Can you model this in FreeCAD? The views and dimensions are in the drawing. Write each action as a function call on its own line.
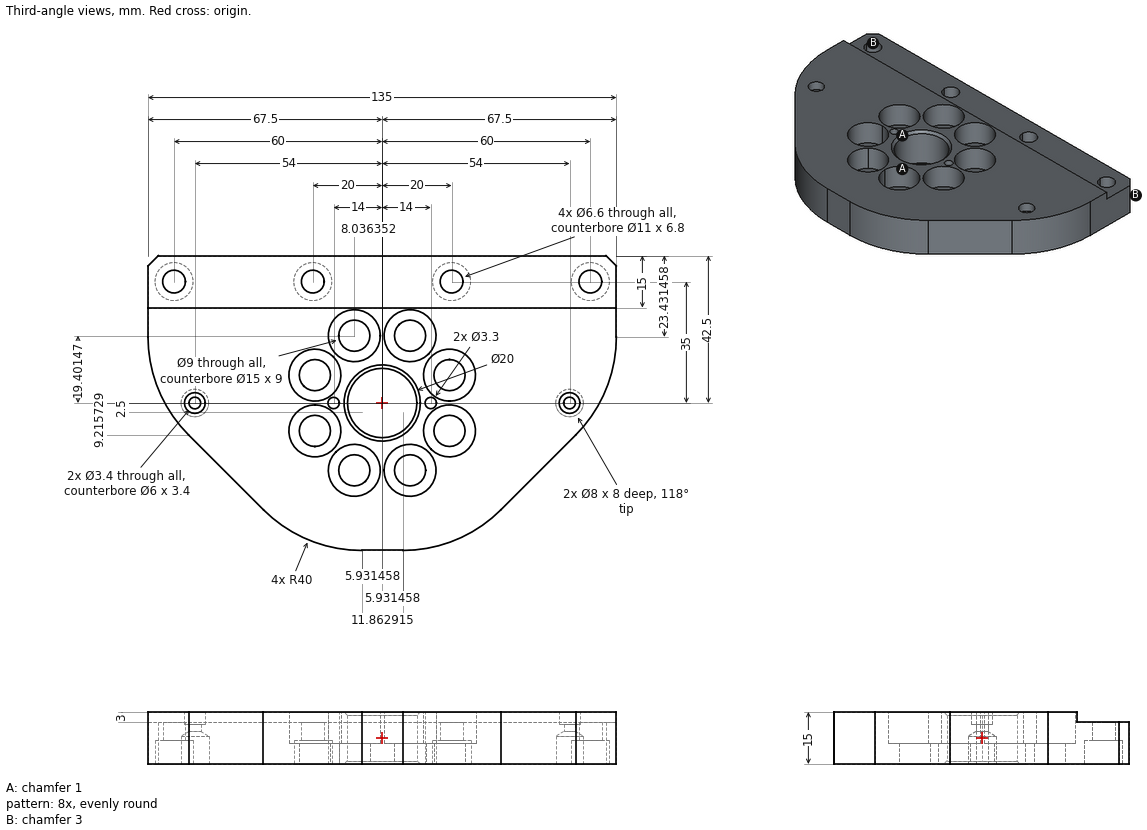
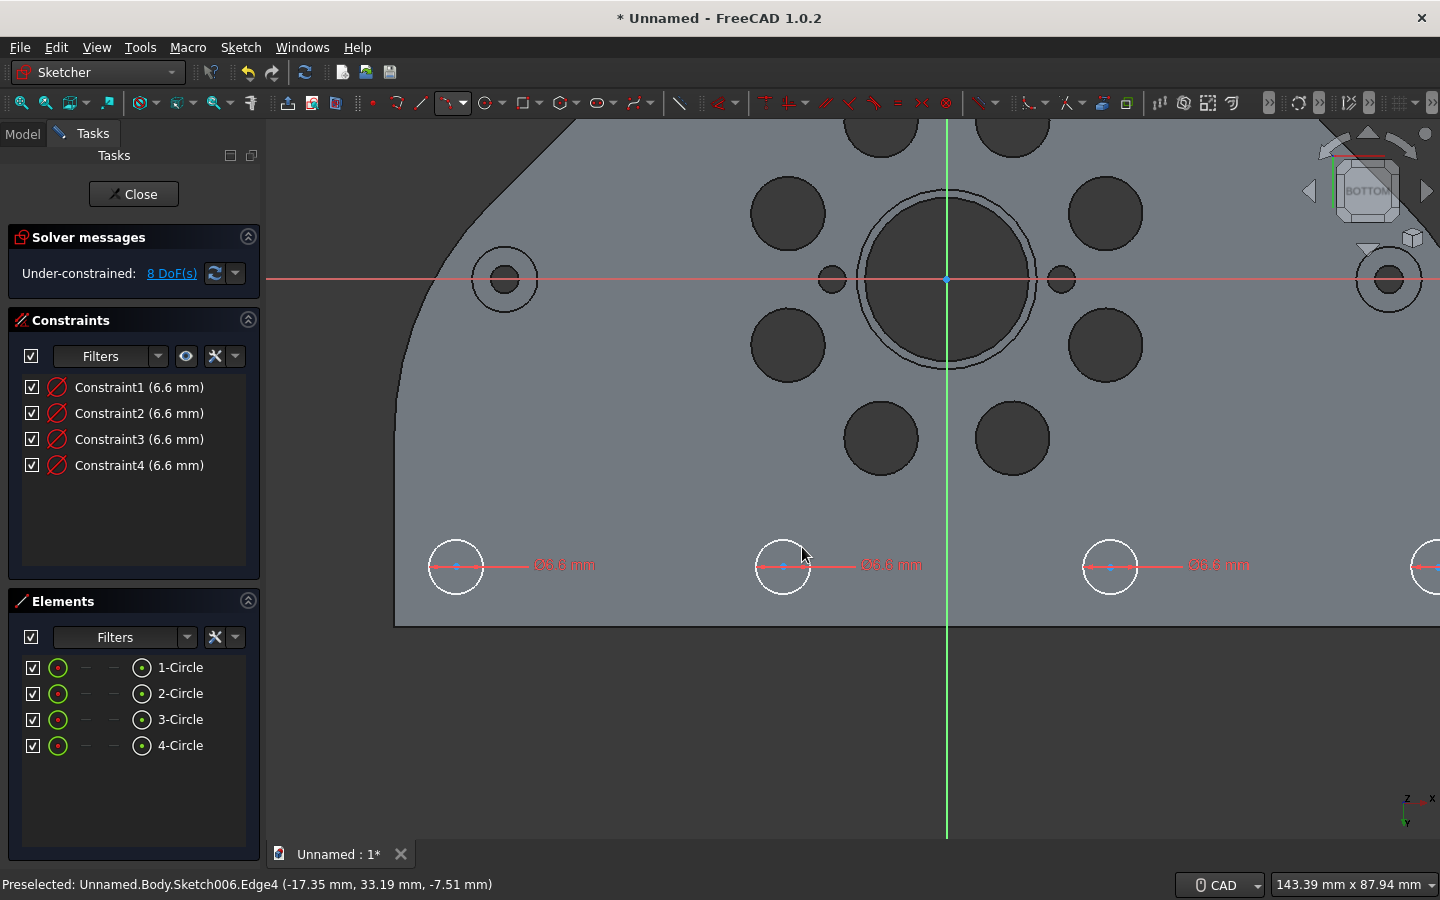
click(1110, 567)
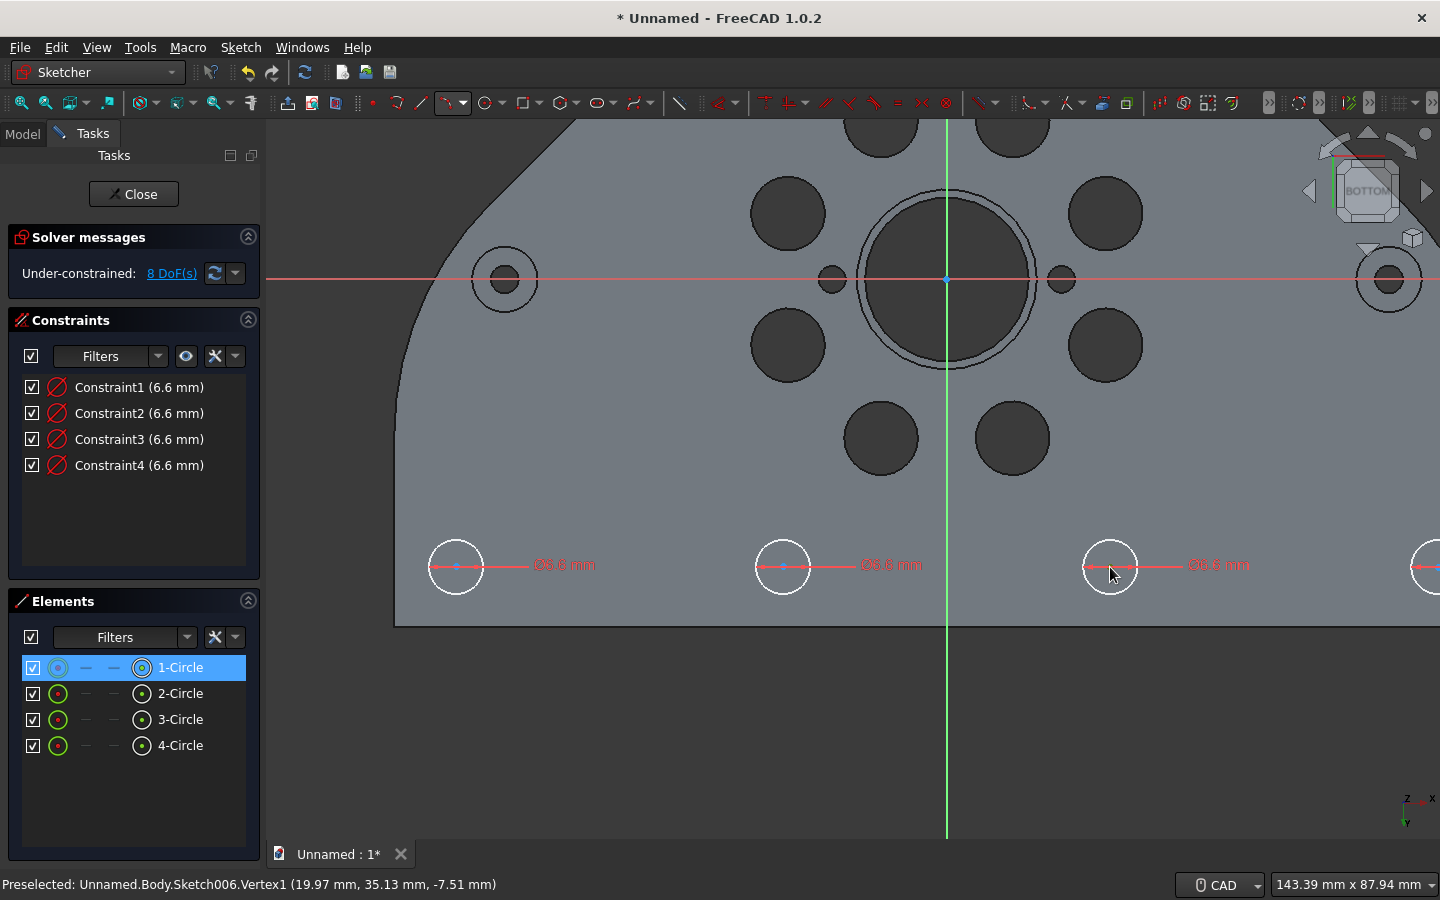
scroll(454, 566, down, 2)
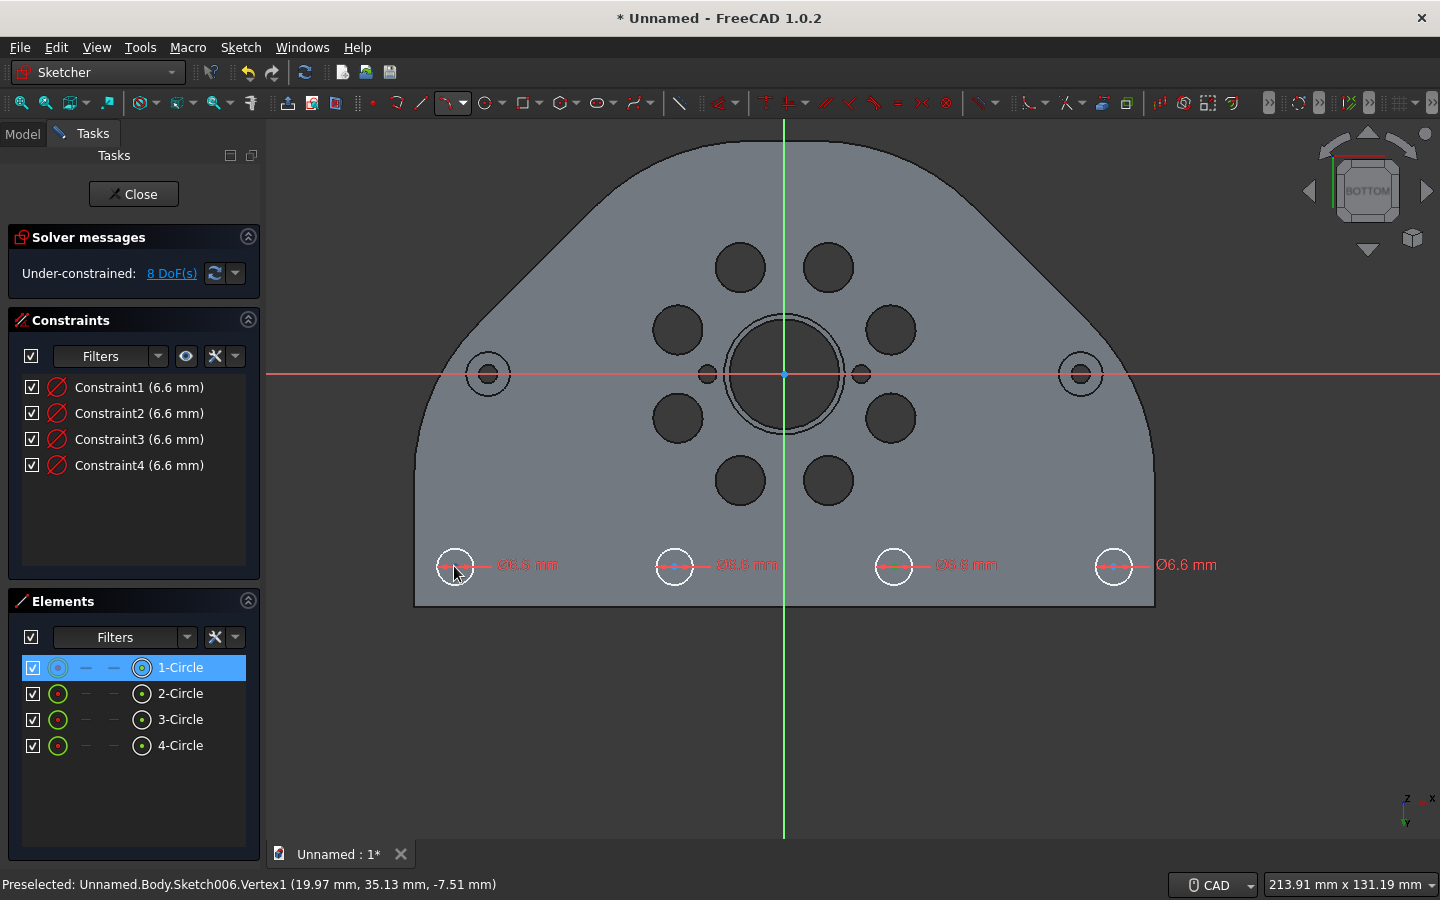
click(1114, 567)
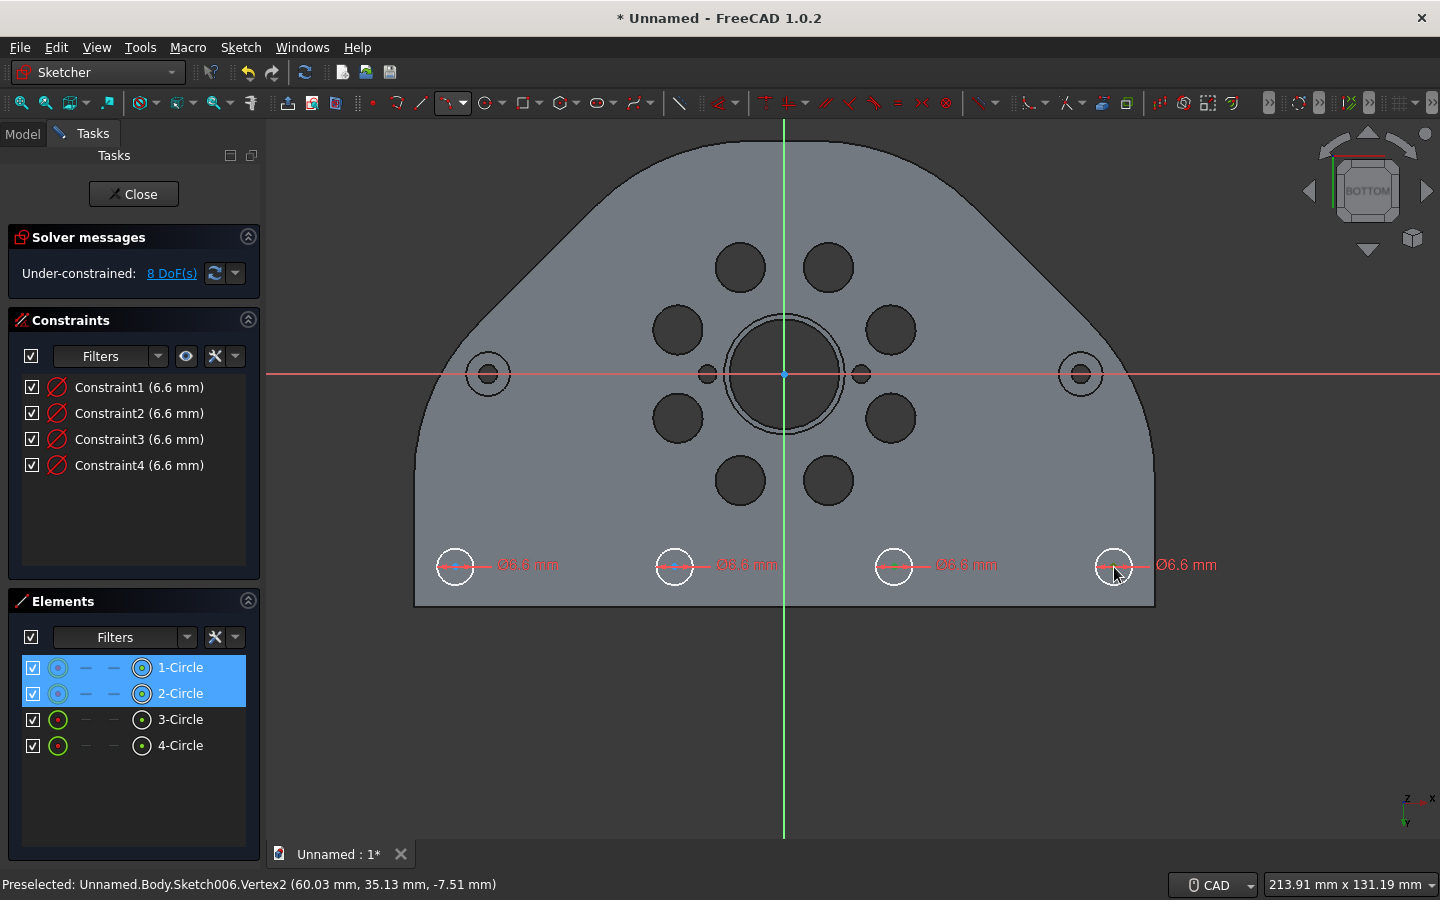
click(808, 104)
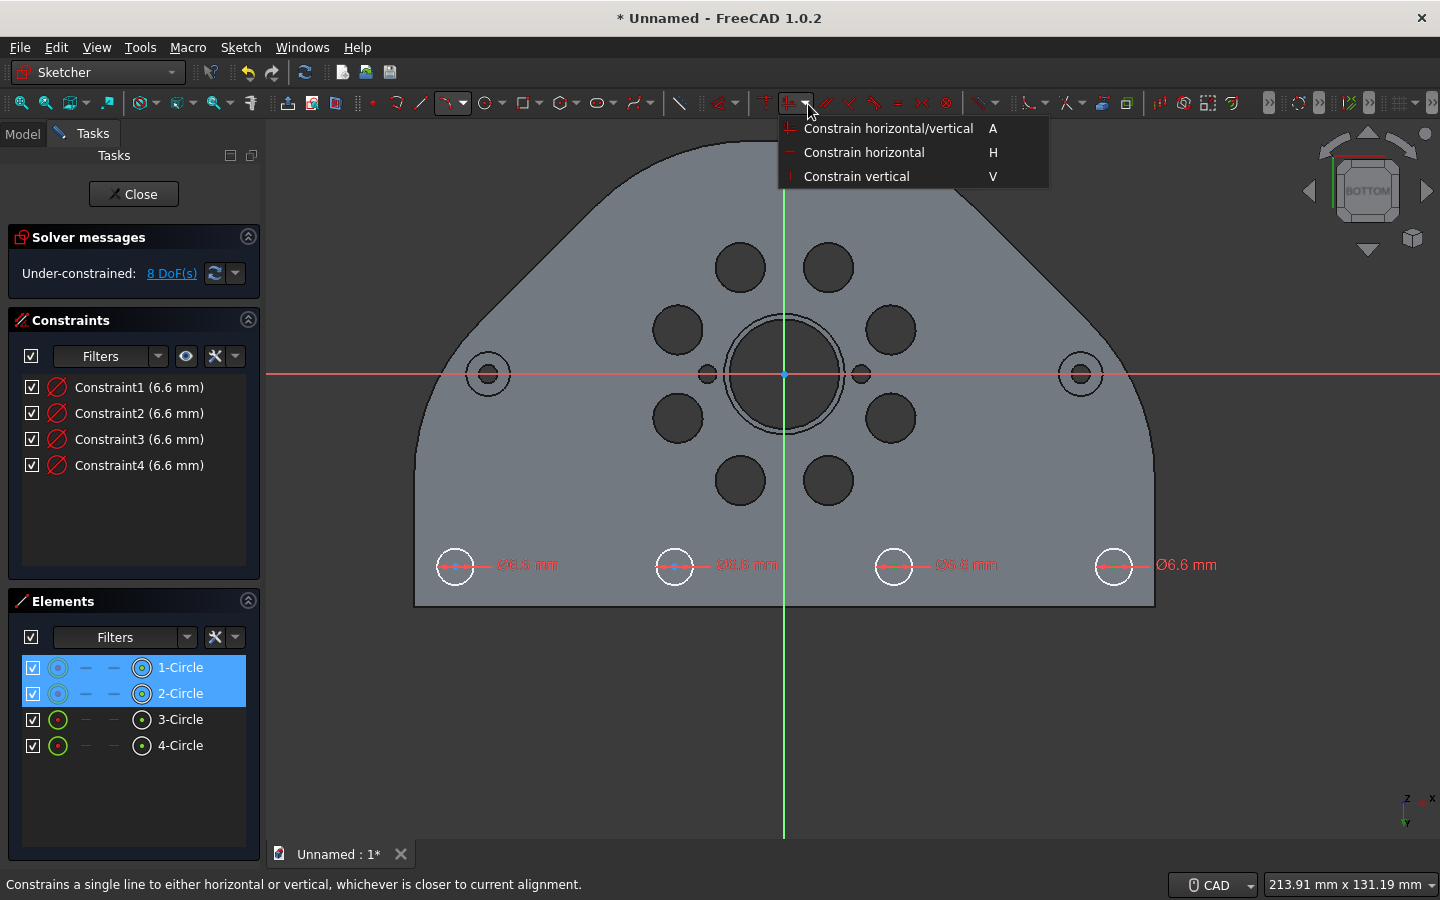
click(914, 152)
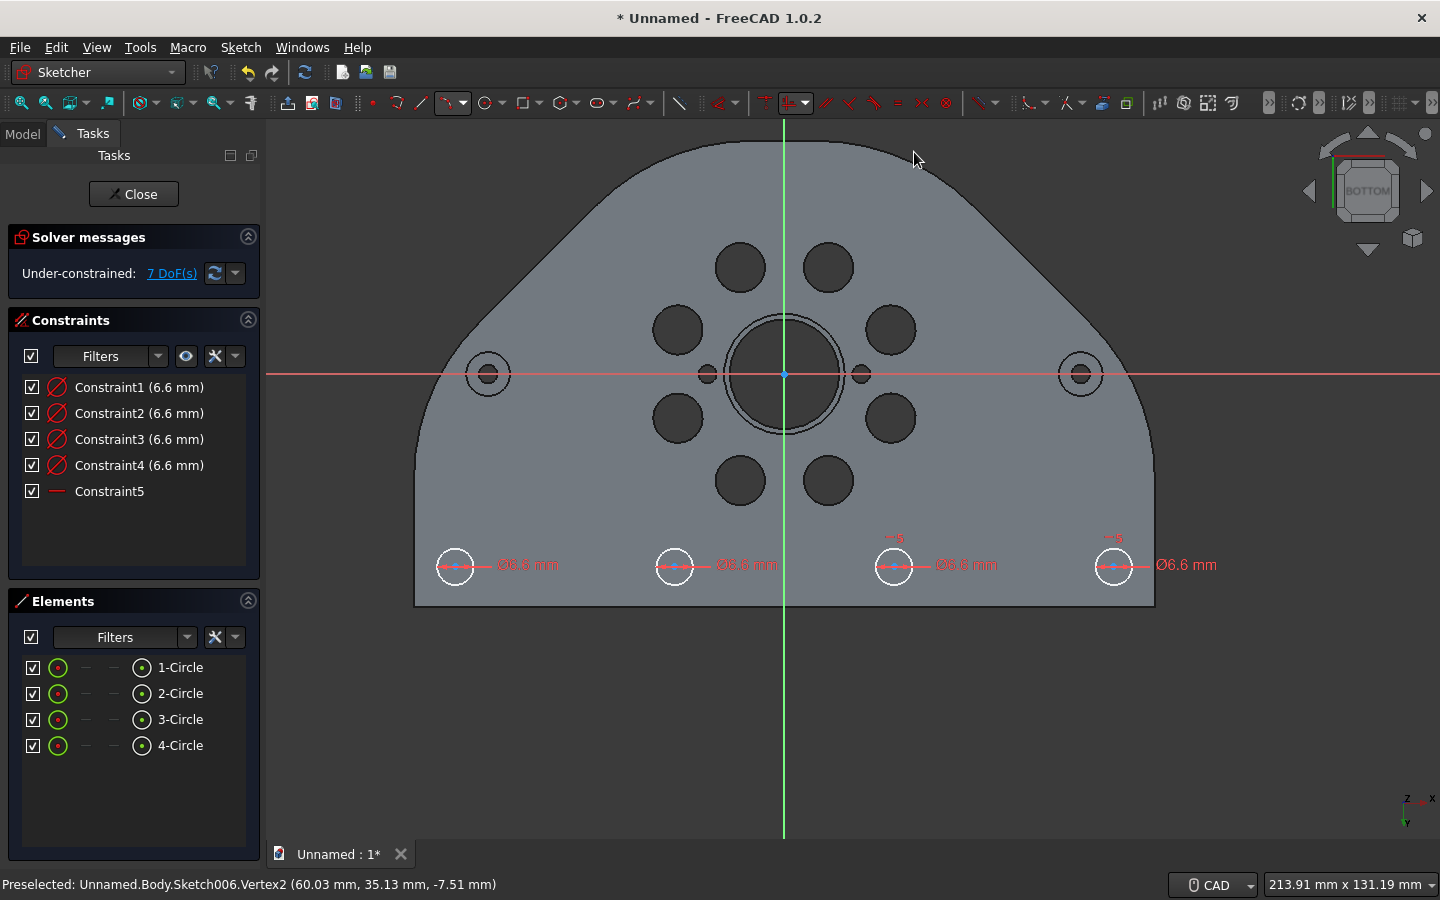
click(894, 567)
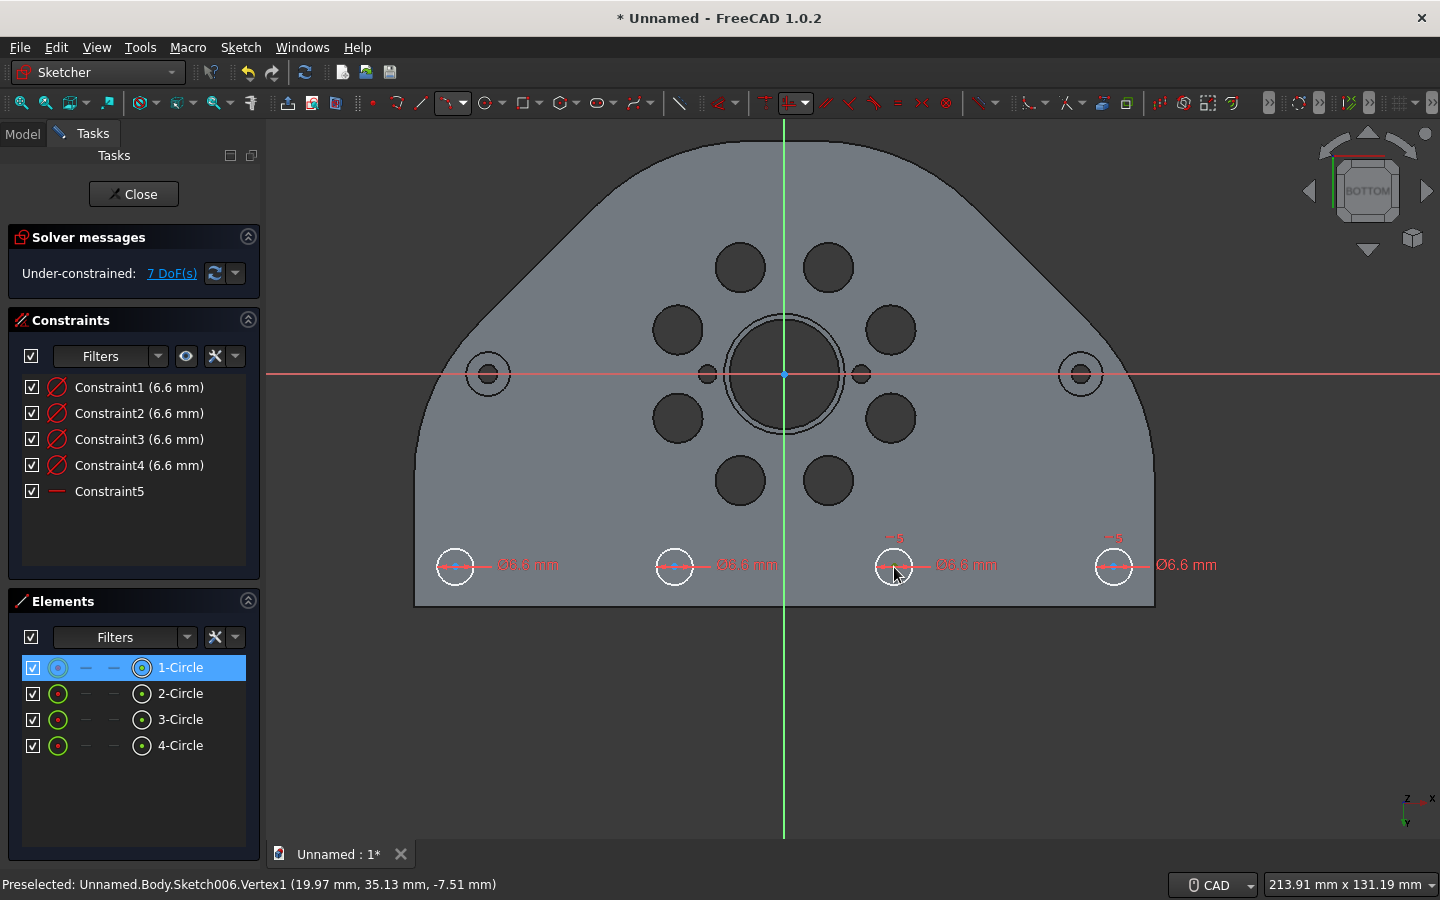
click(455, 567)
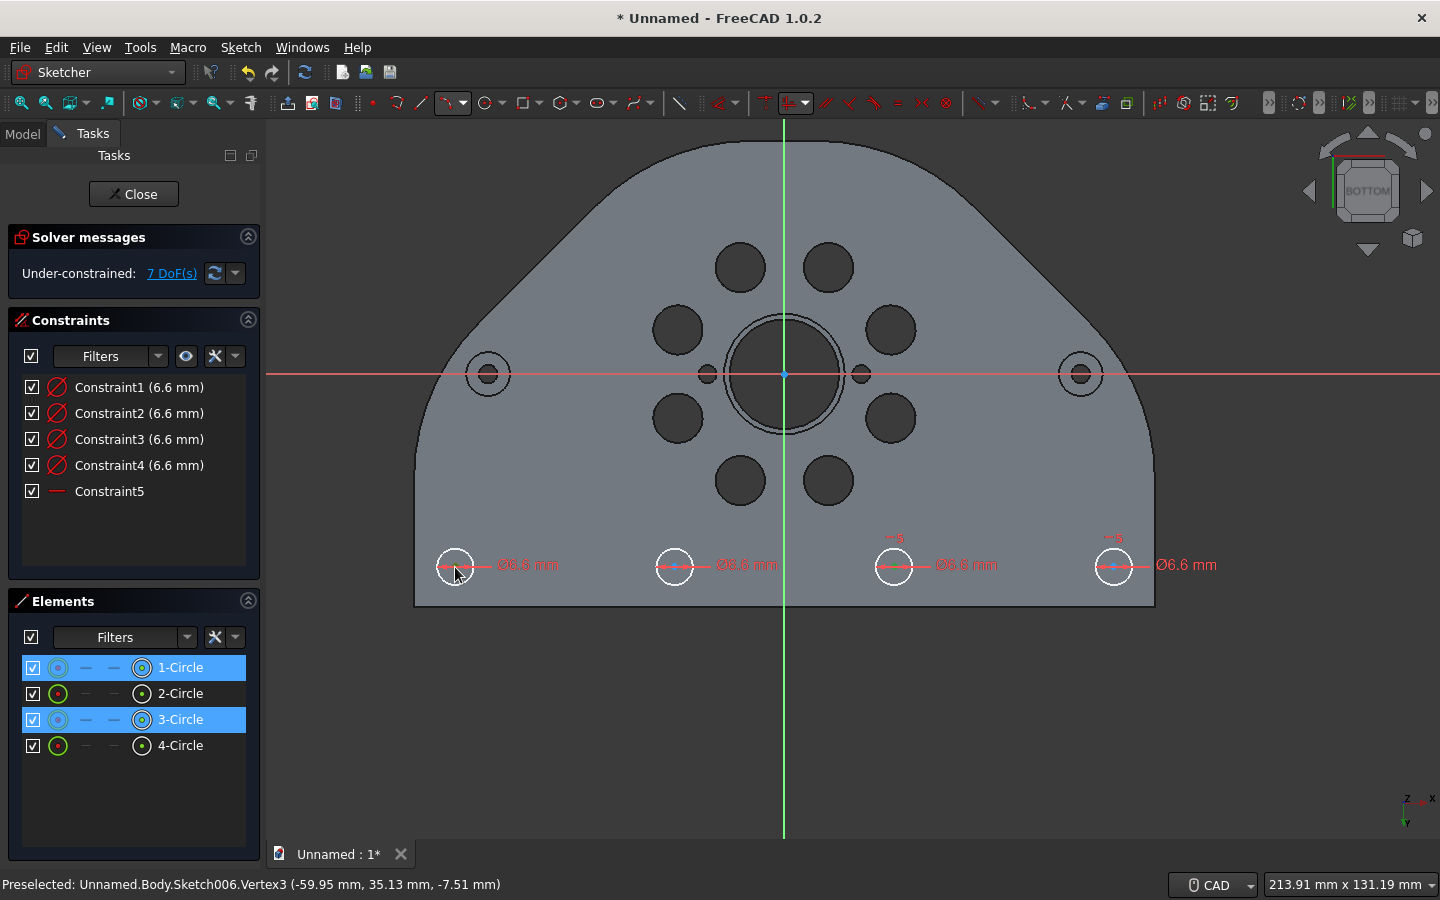
key(h)